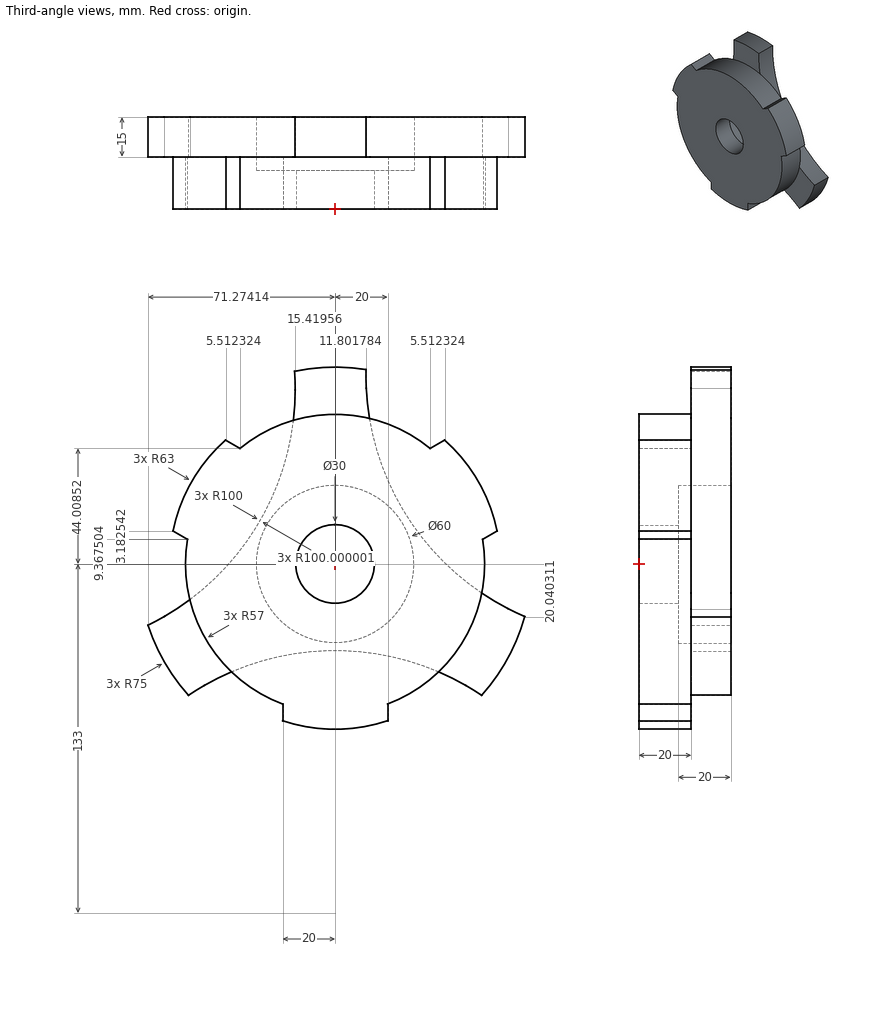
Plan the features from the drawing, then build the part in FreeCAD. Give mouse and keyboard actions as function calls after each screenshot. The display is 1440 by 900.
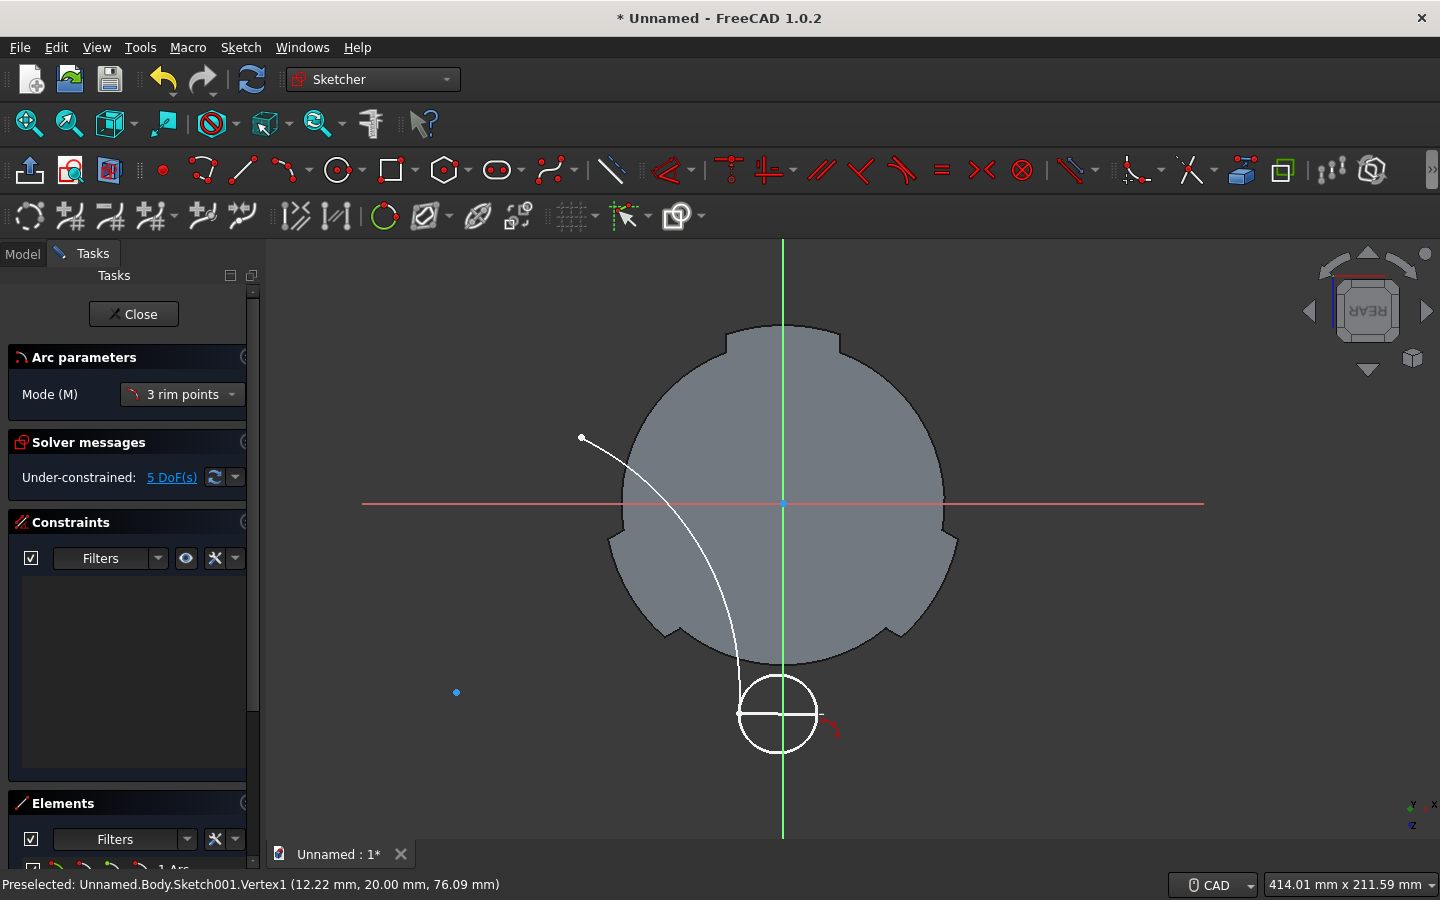
scroll(778, 716, up, 8)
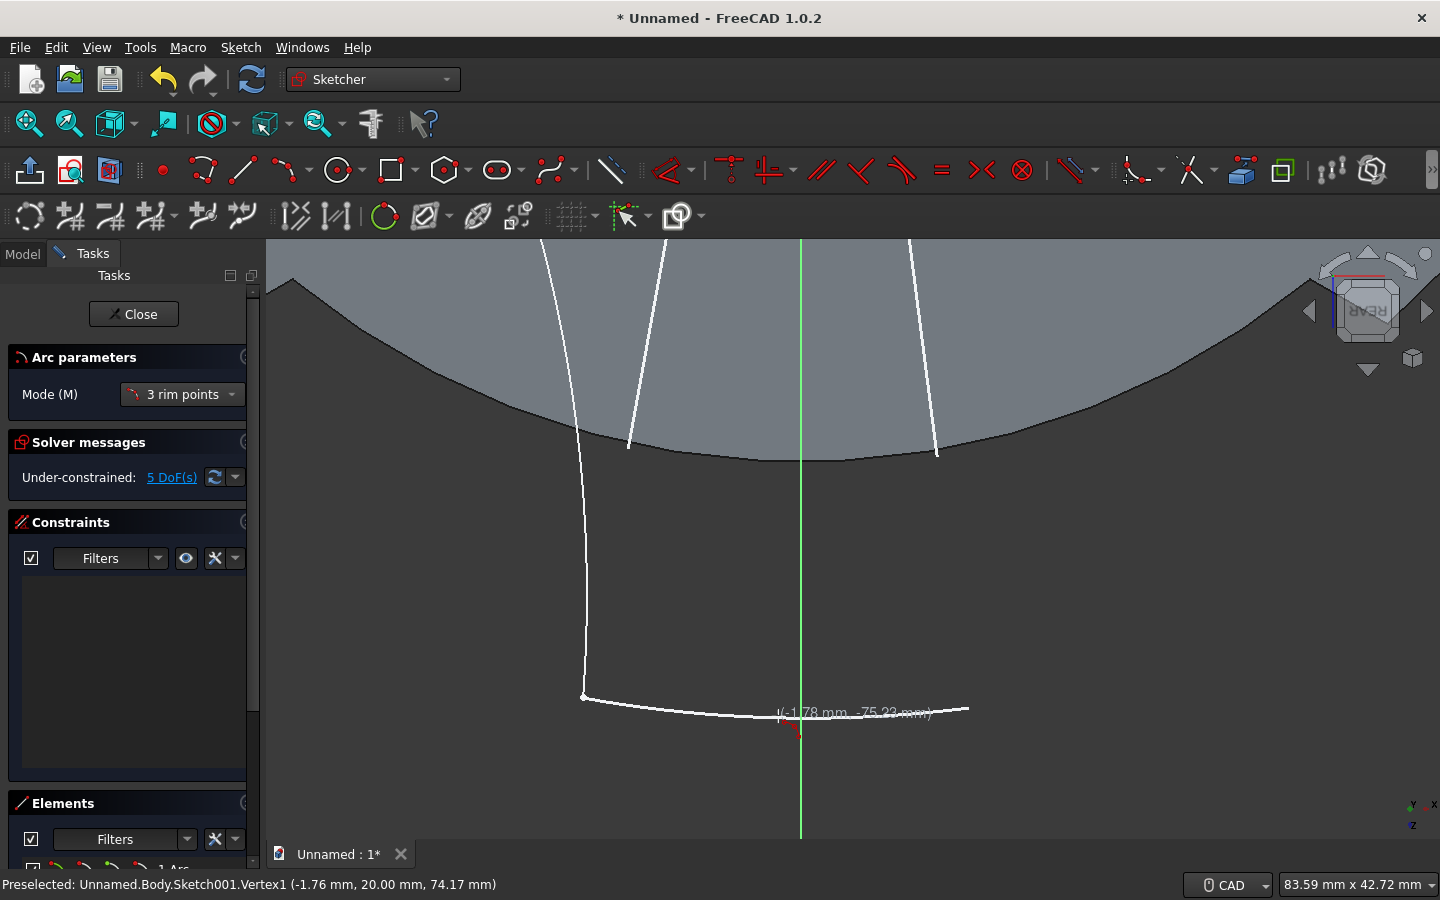
click(776, 714)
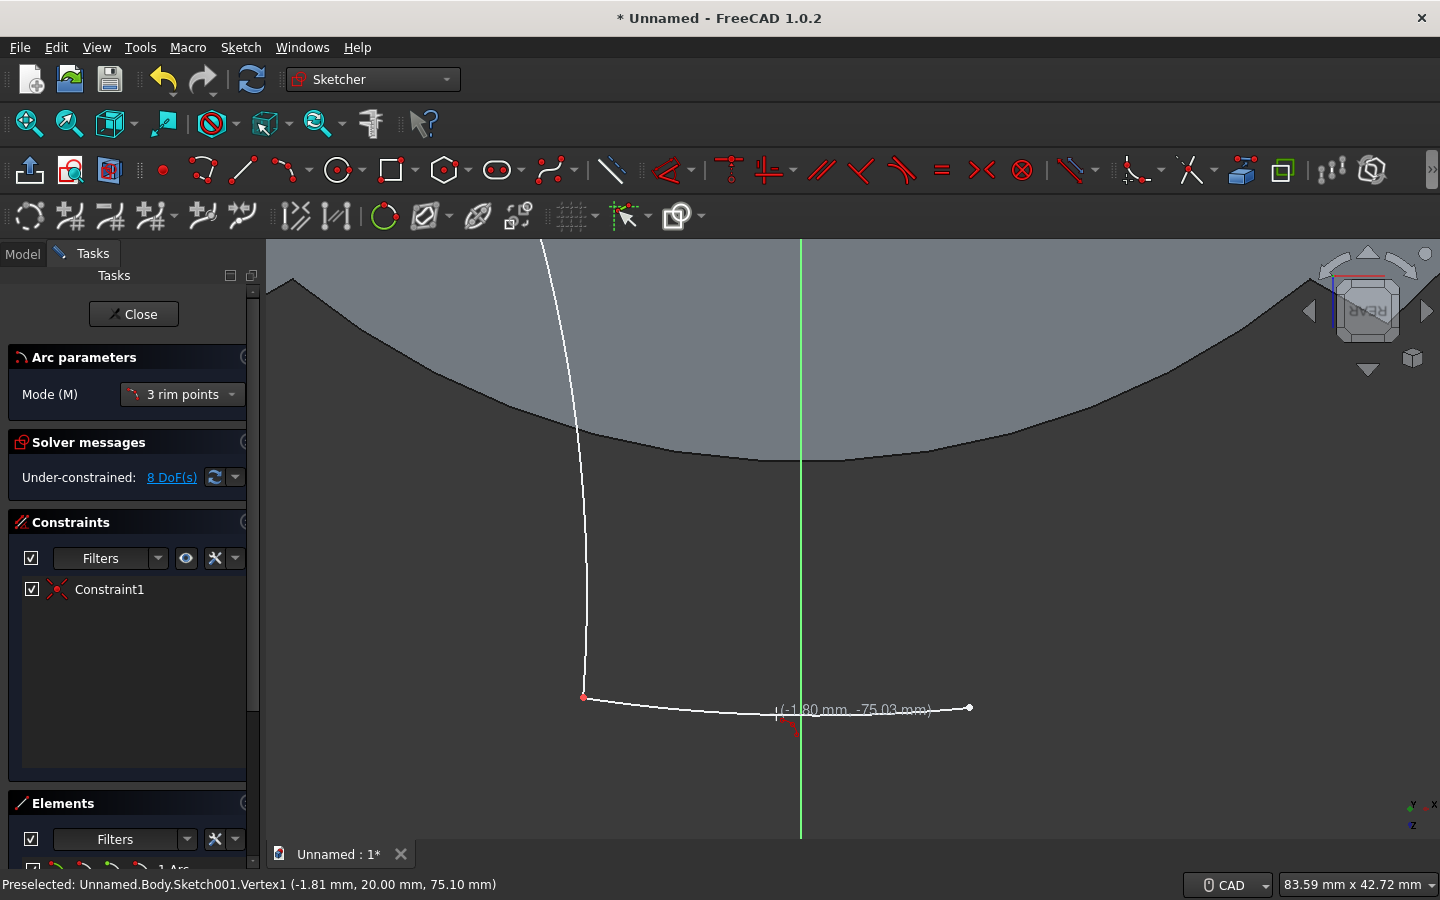
scroll(778, 717, down, 8)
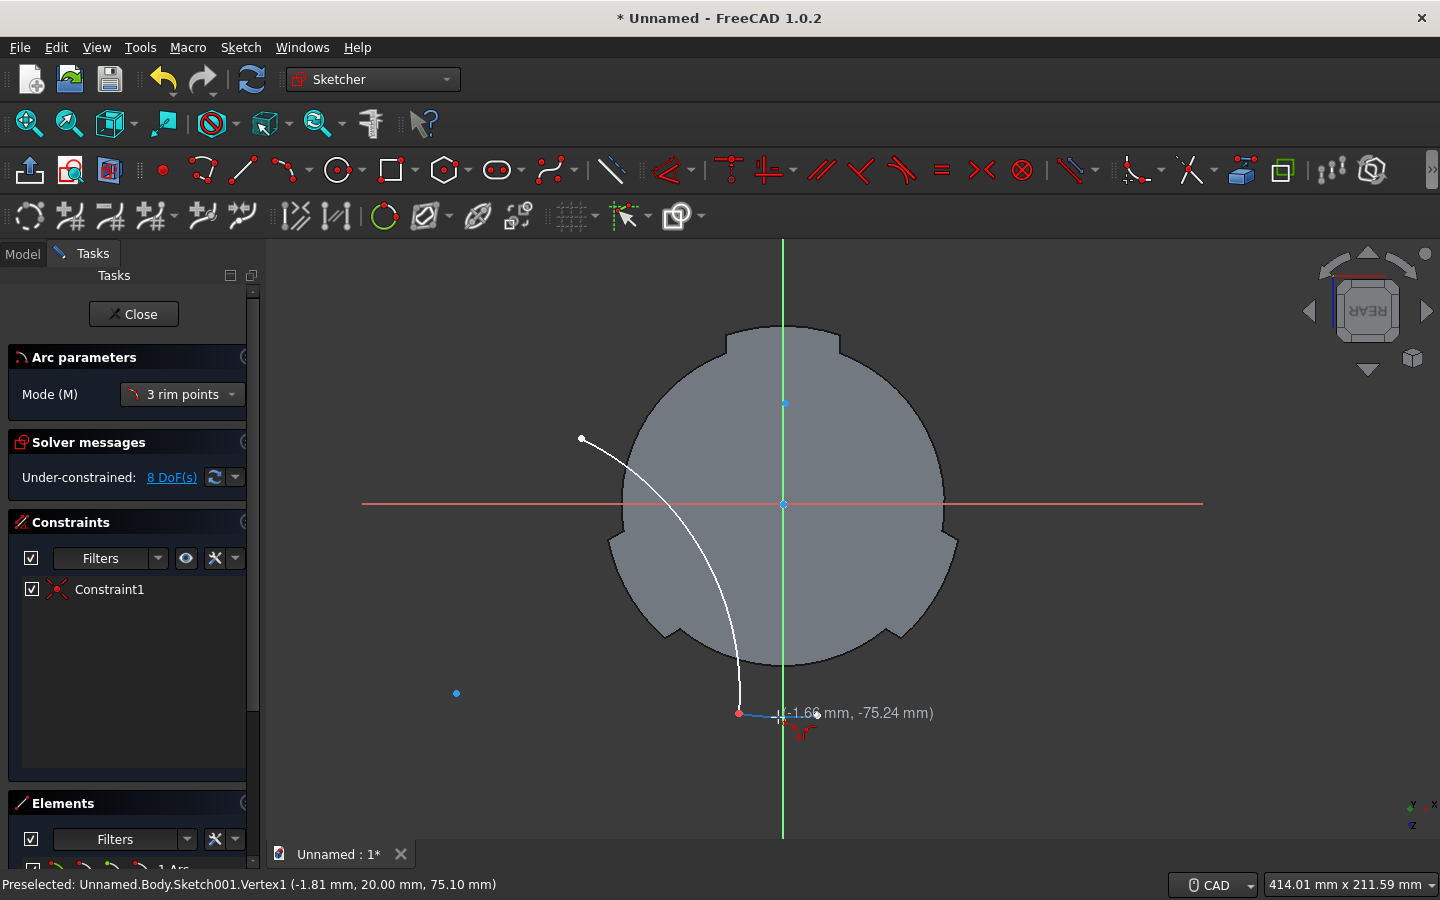
click(817, 716)
click(988, 448)
click(861, 555)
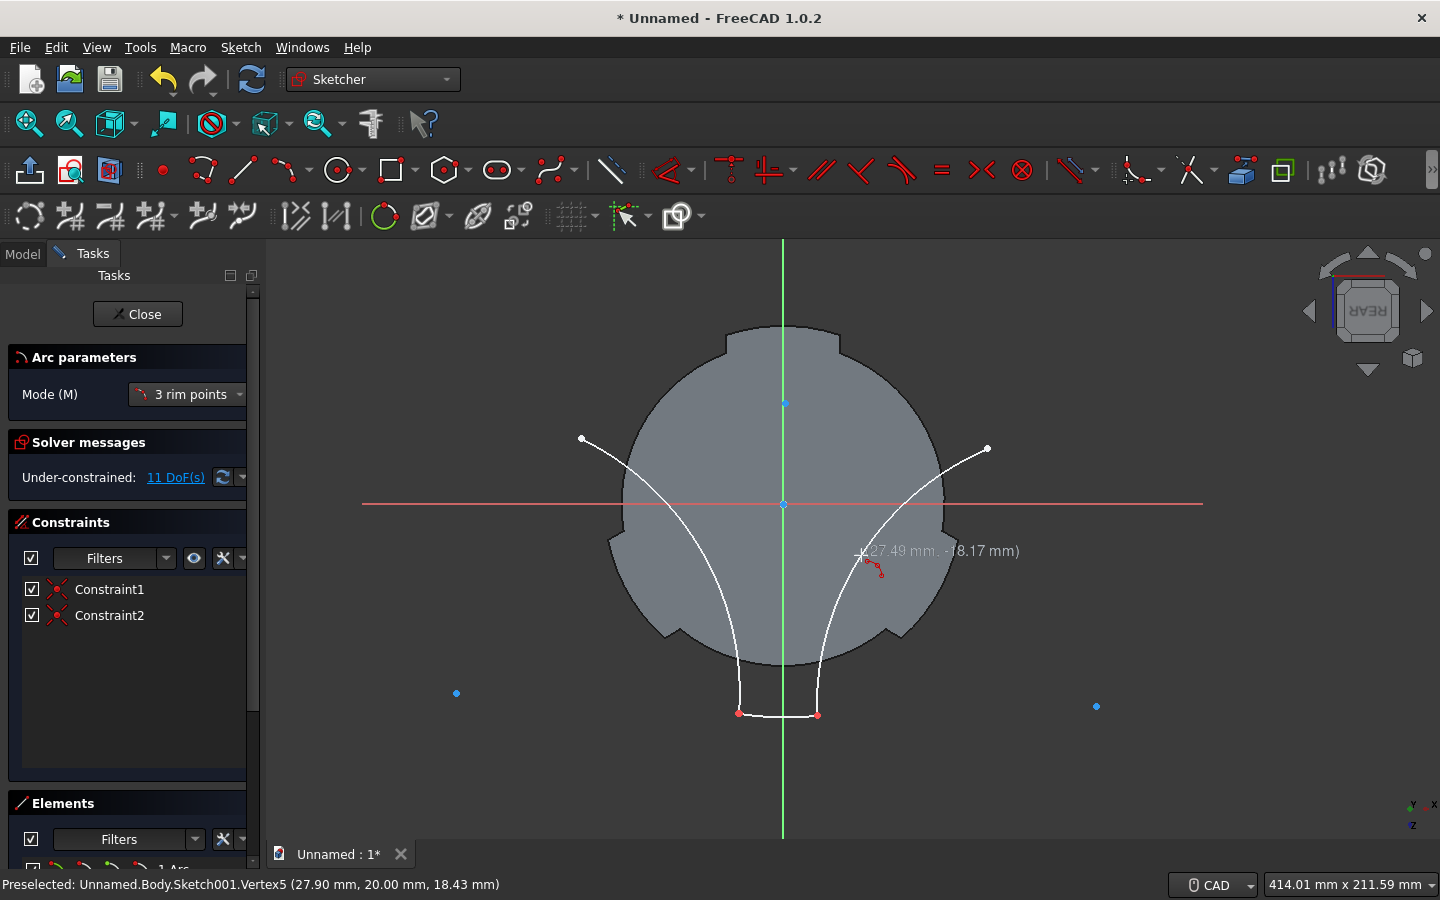
click(988, 449)
click(941, 363)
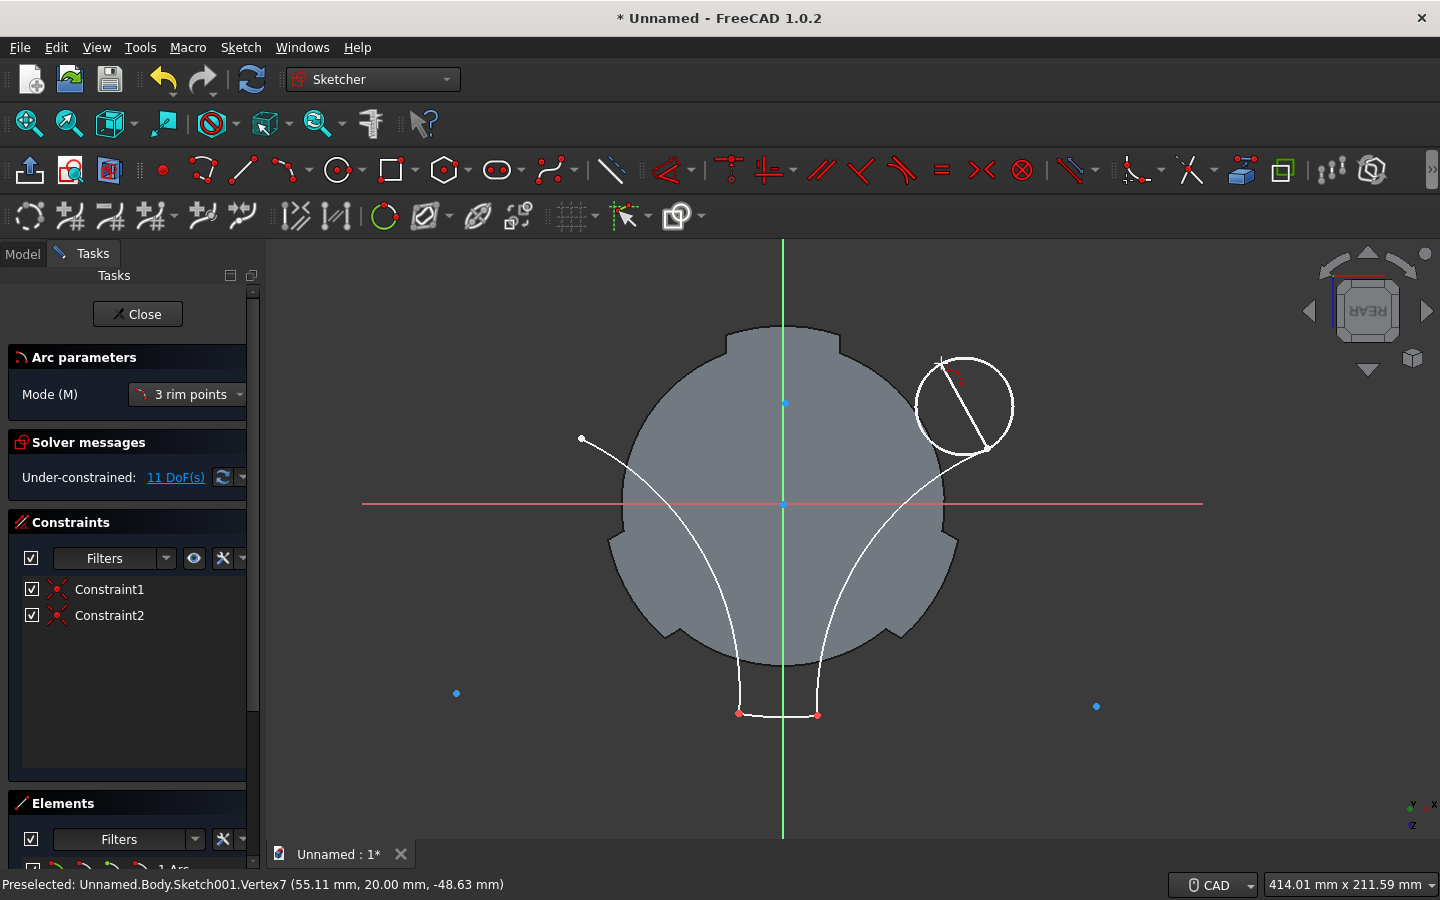
scroll(970, 402, up, 6)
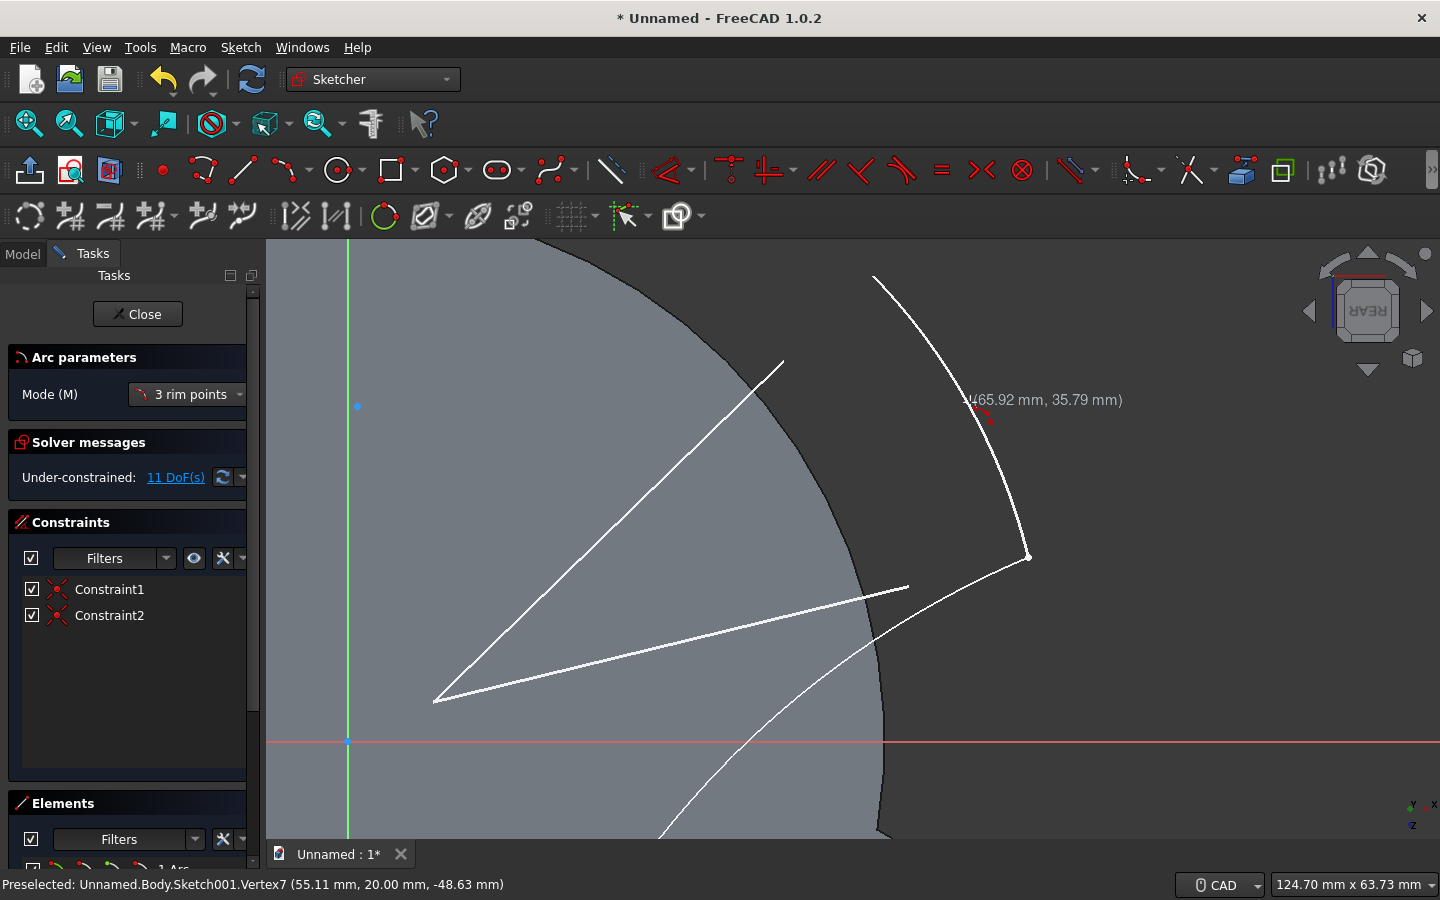
click(967, 403)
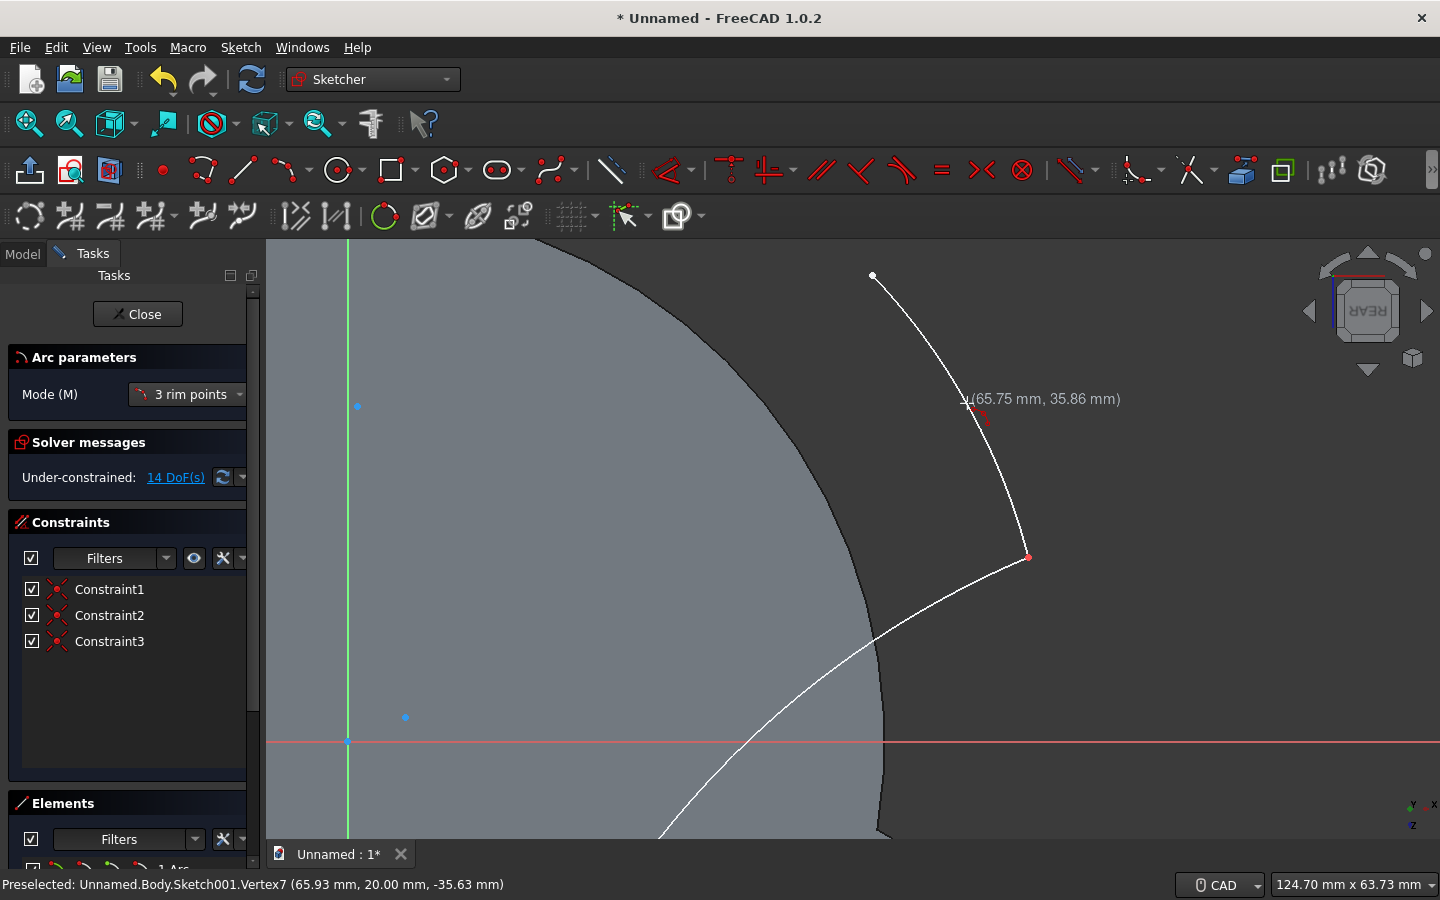
click(872, 275)